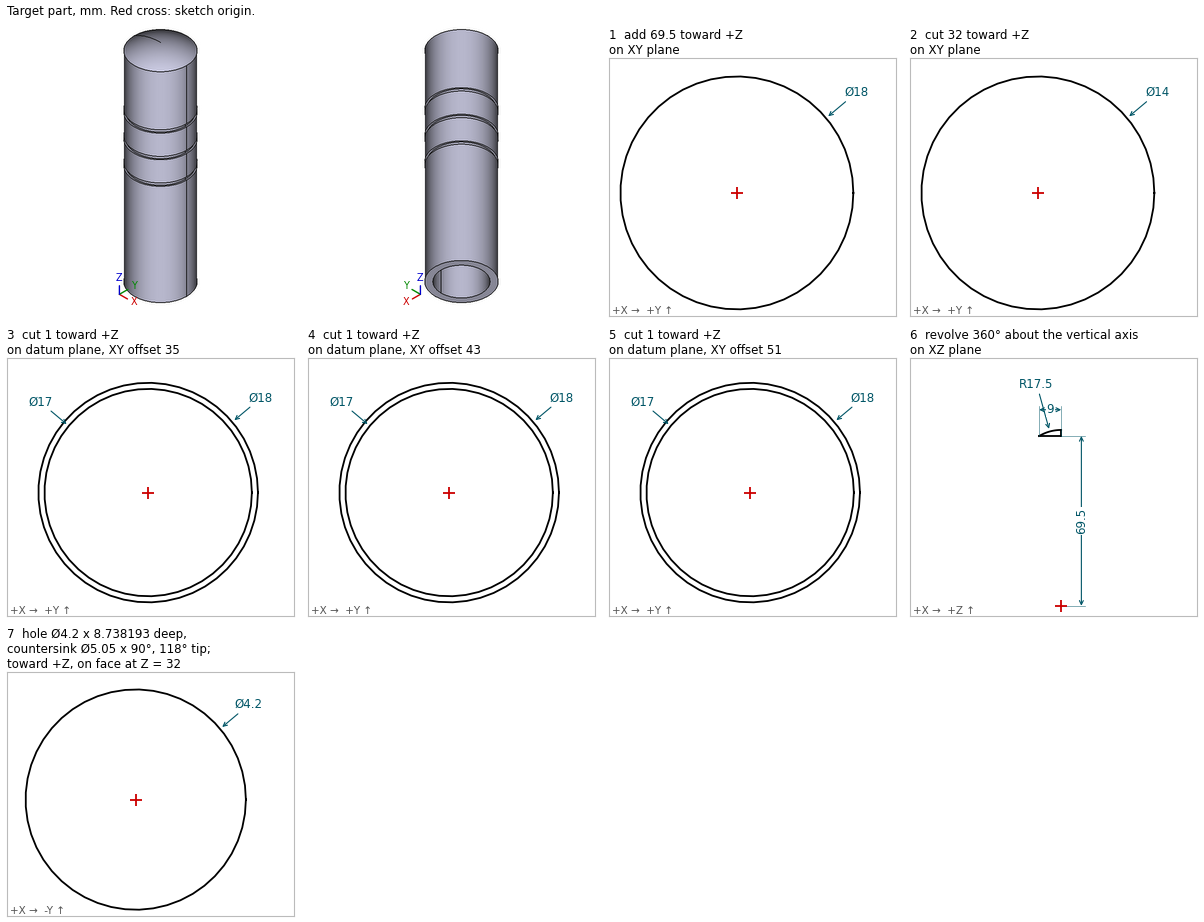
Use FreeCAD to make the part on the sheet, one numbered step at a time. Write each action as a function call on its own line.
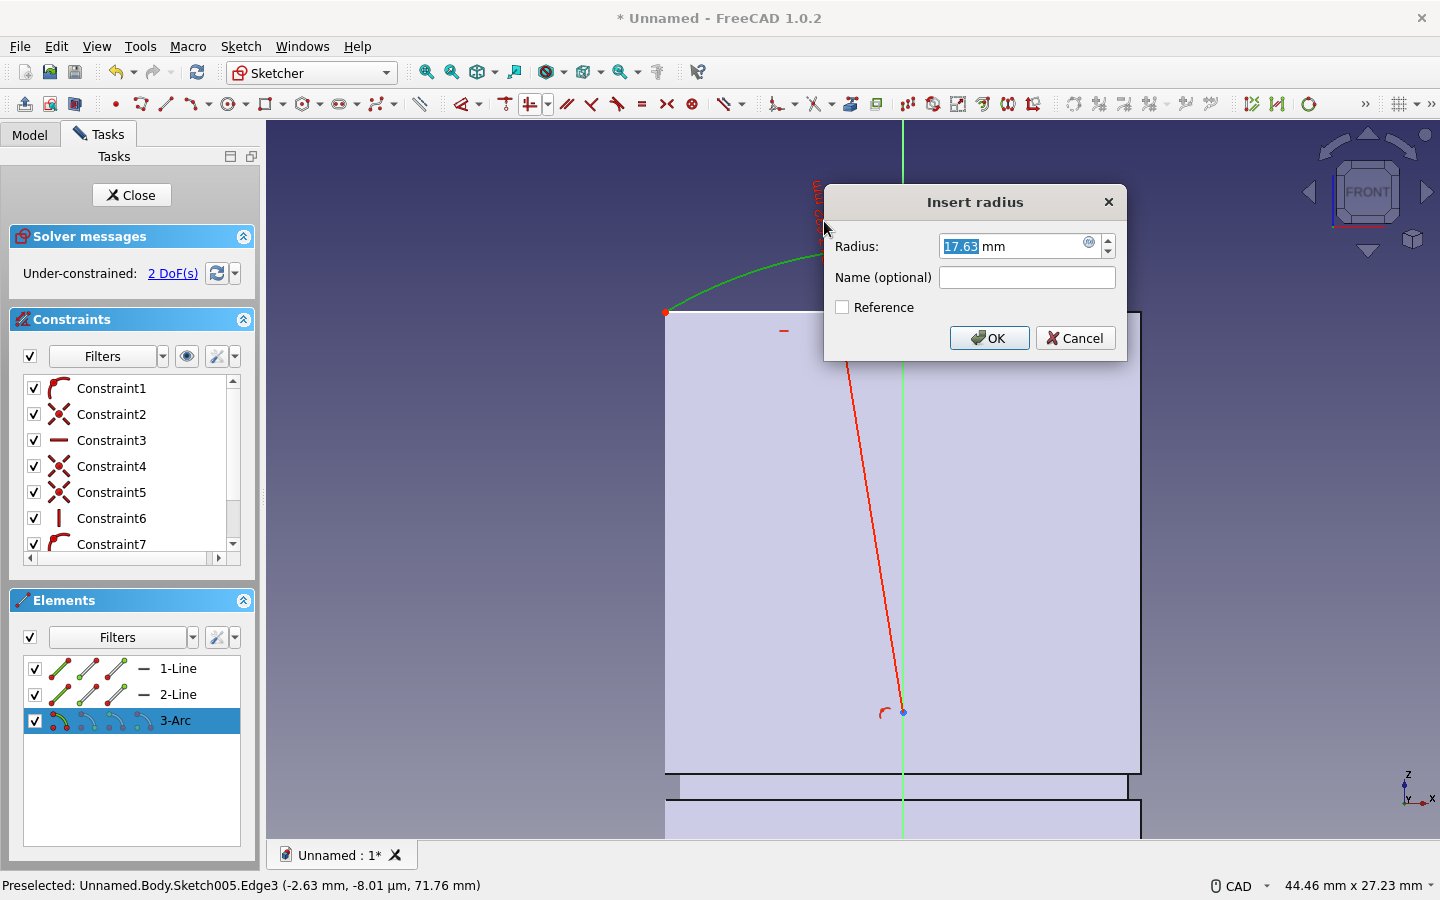
text(17.5)
key(Return)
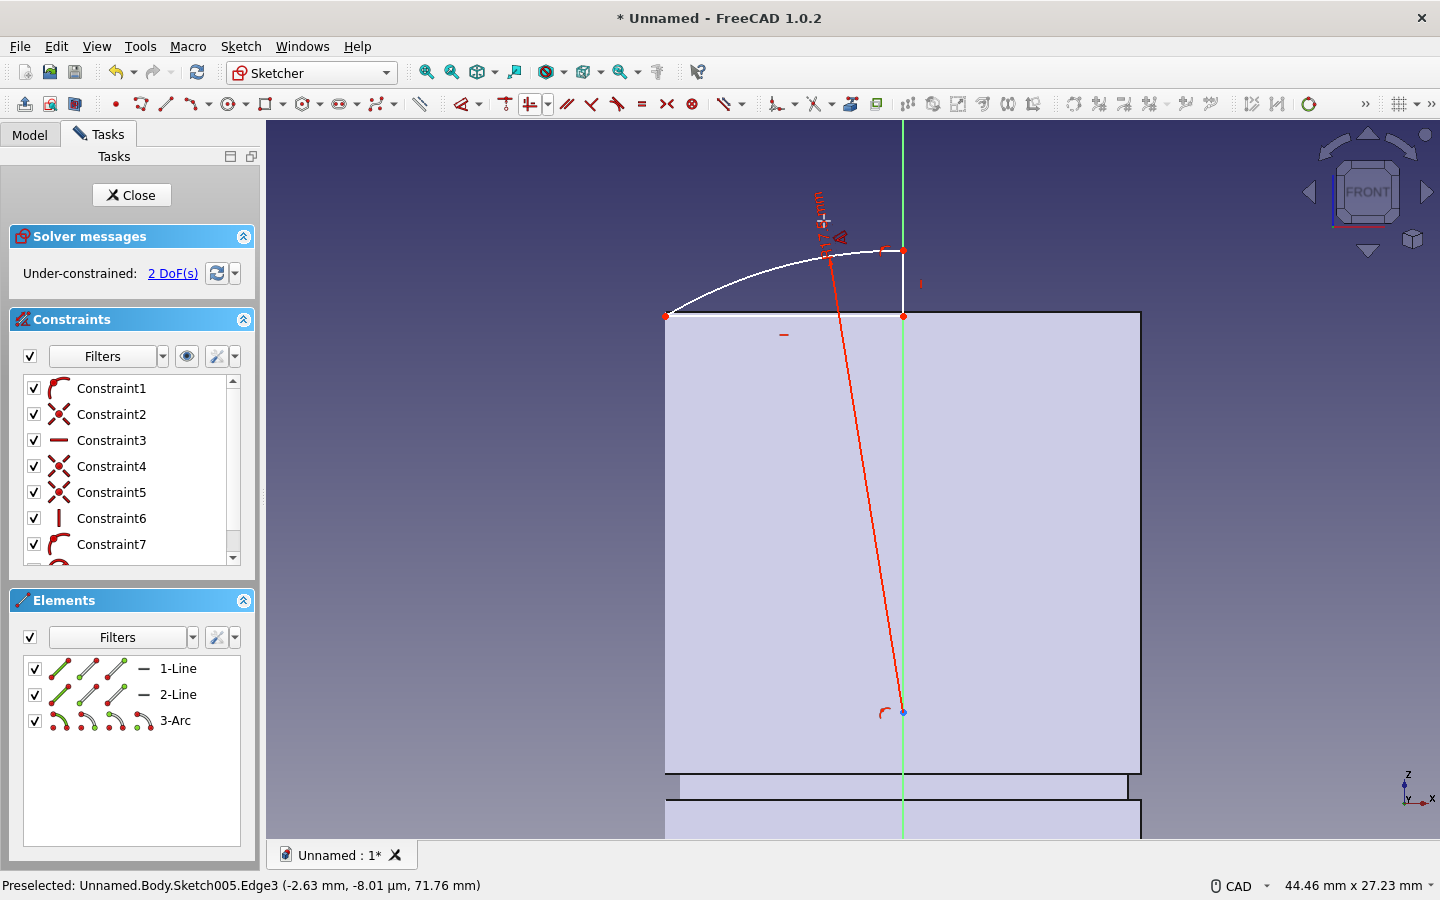
click(832, 316)
click(784, 350)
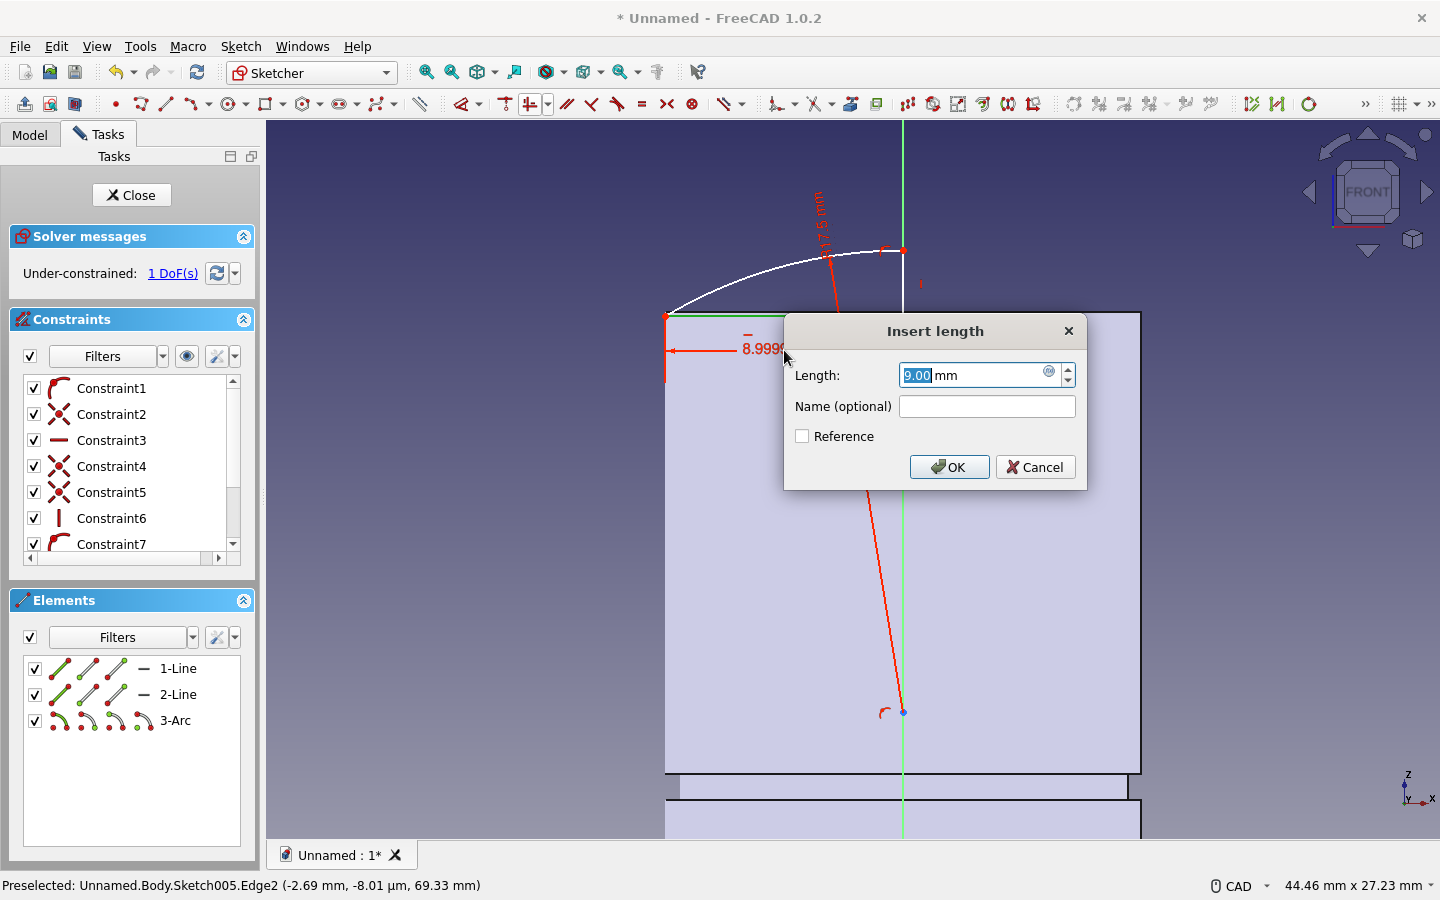
text(9)
key(Return)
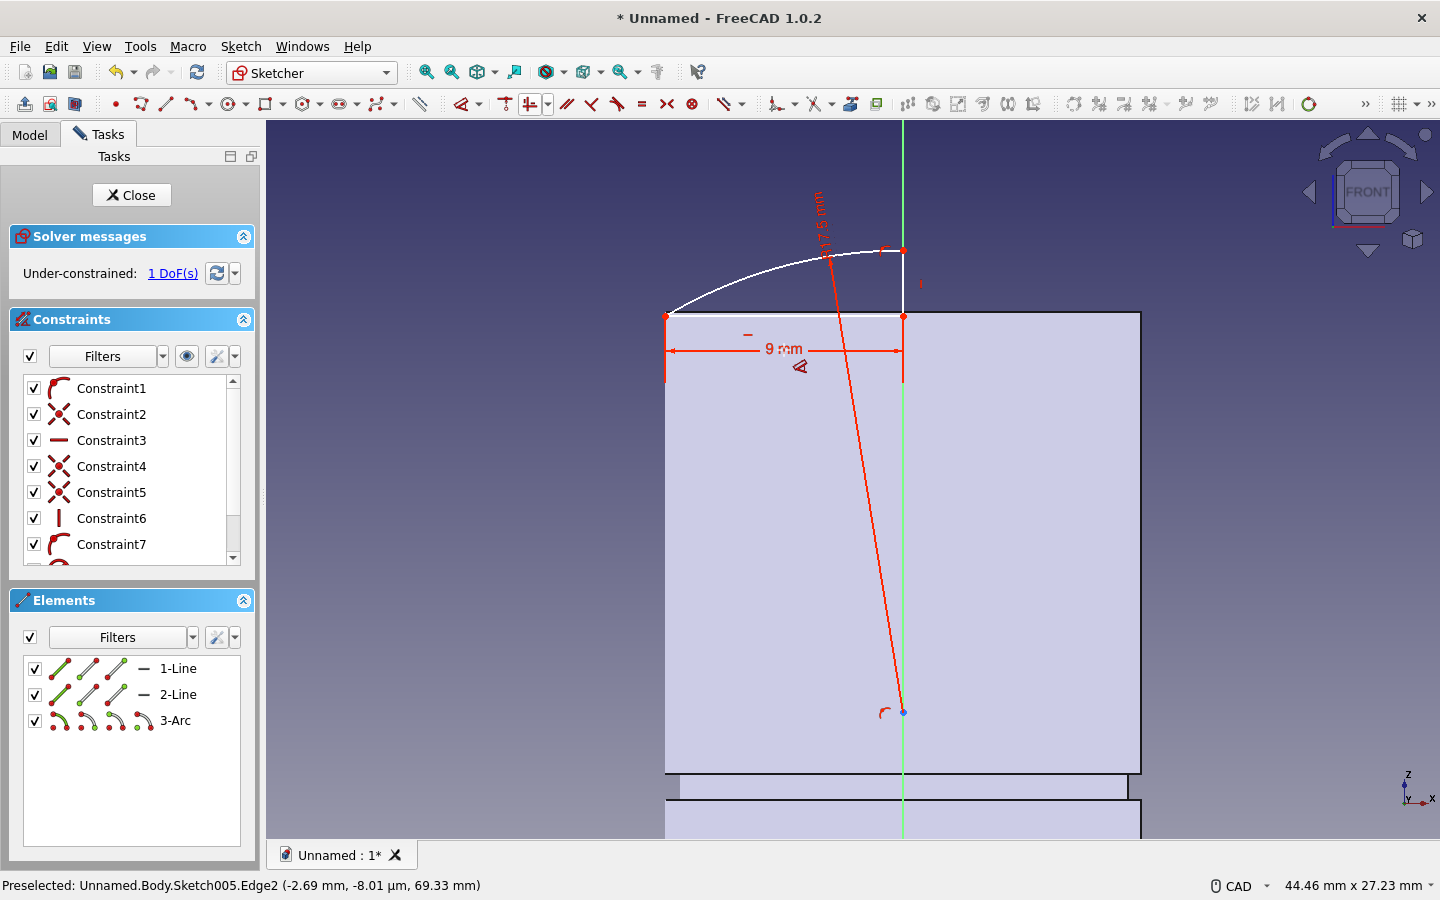
click(903, 316)
click(937, 564)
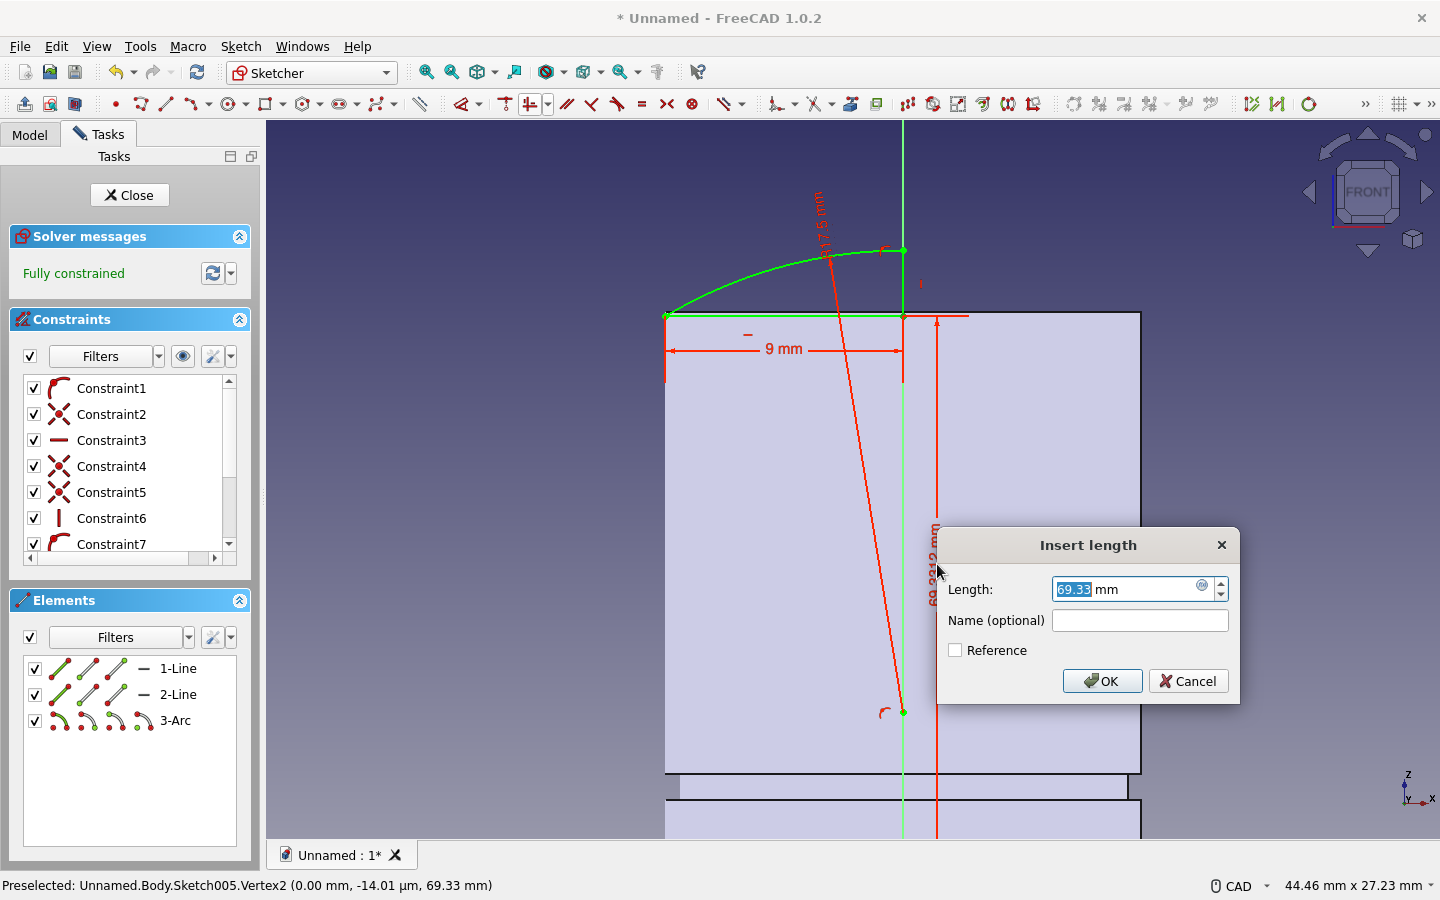
text(69.5)
key(Return)
key(Escape)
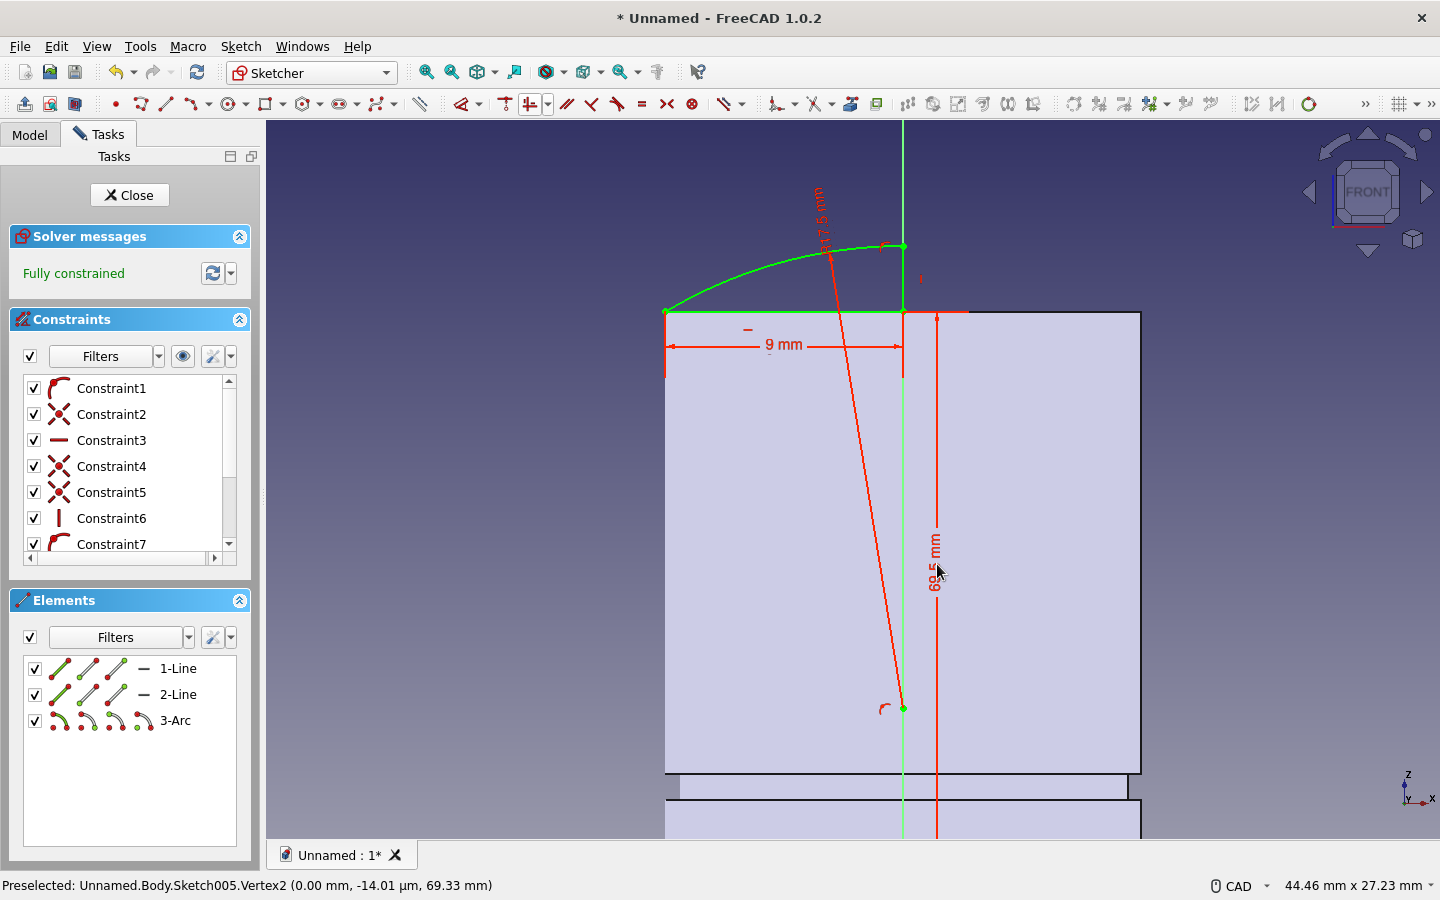
click(130, 195)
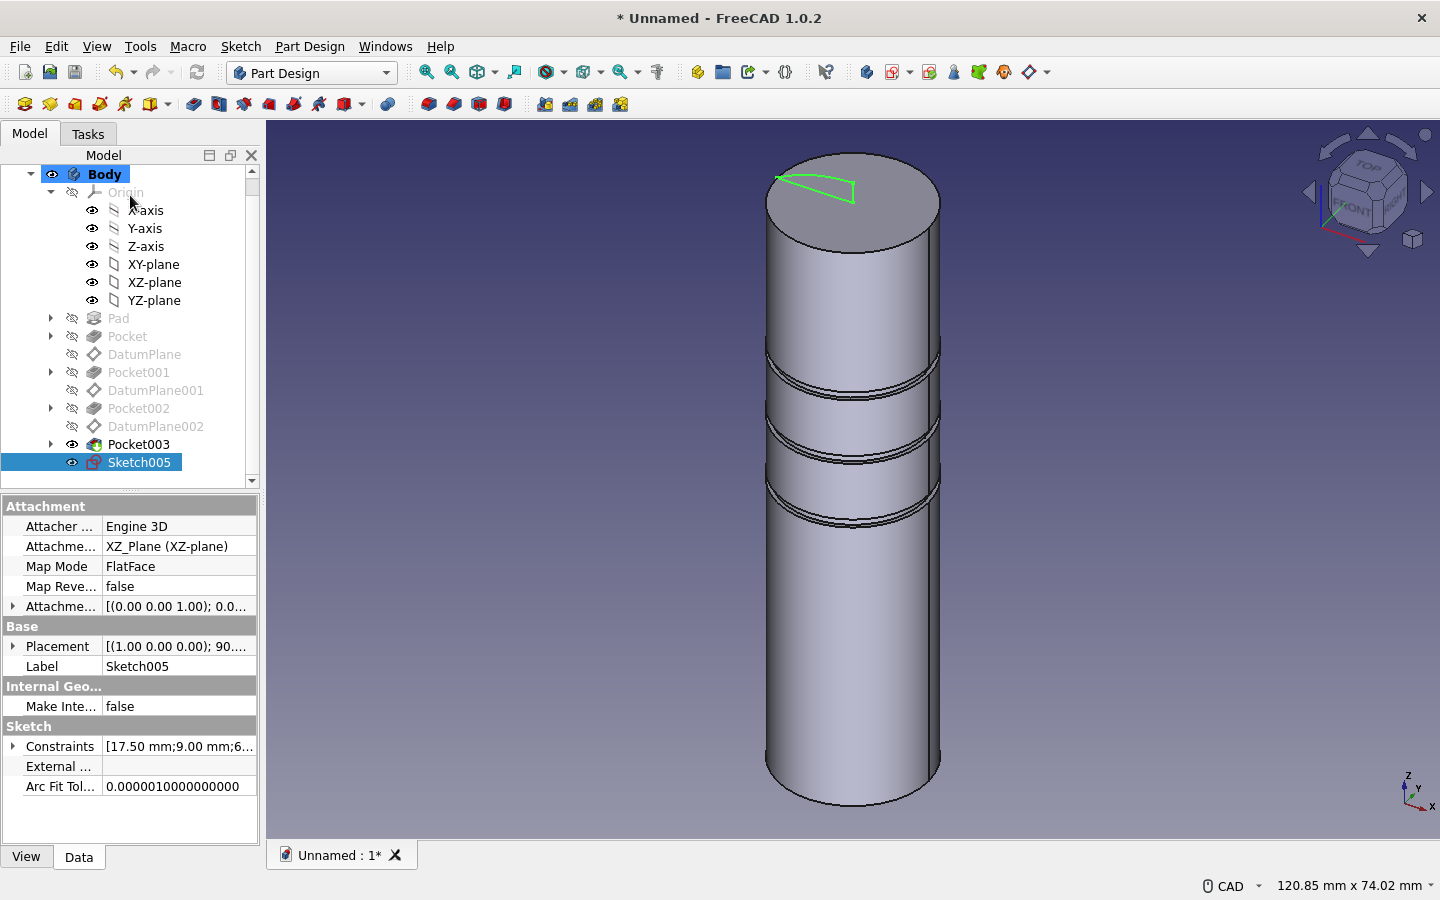
click(50, 104)